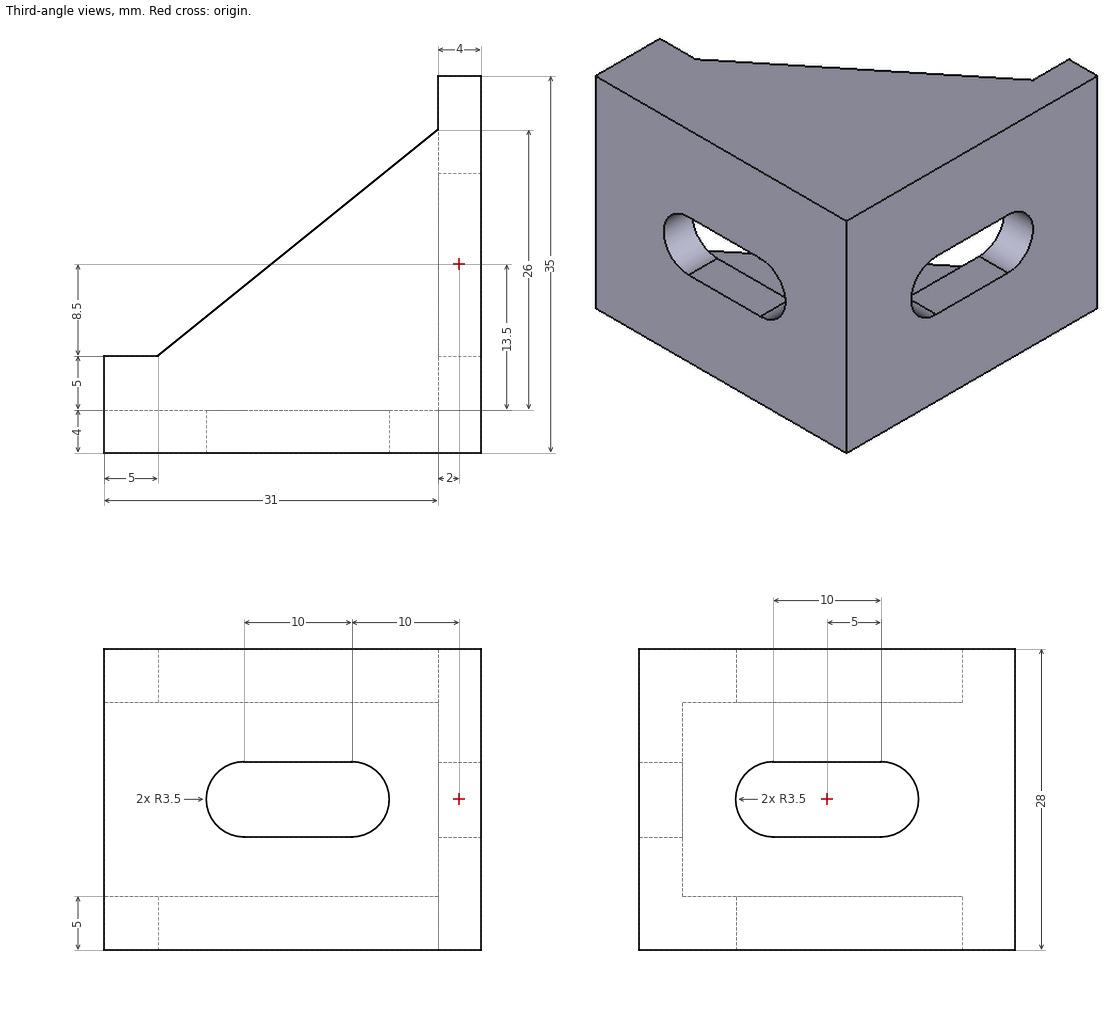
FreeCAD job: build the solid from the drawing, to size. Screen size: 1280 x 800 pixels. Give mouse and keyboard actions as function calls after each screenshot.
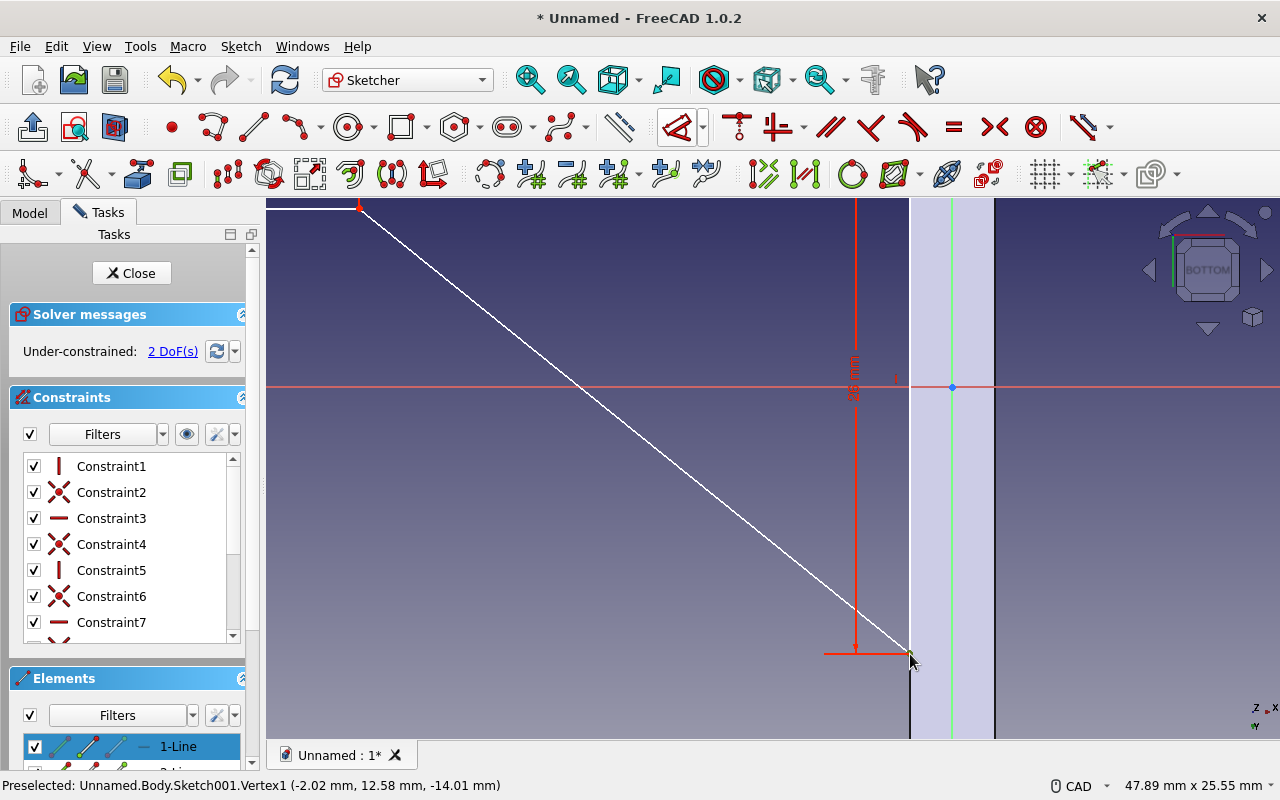
key(l)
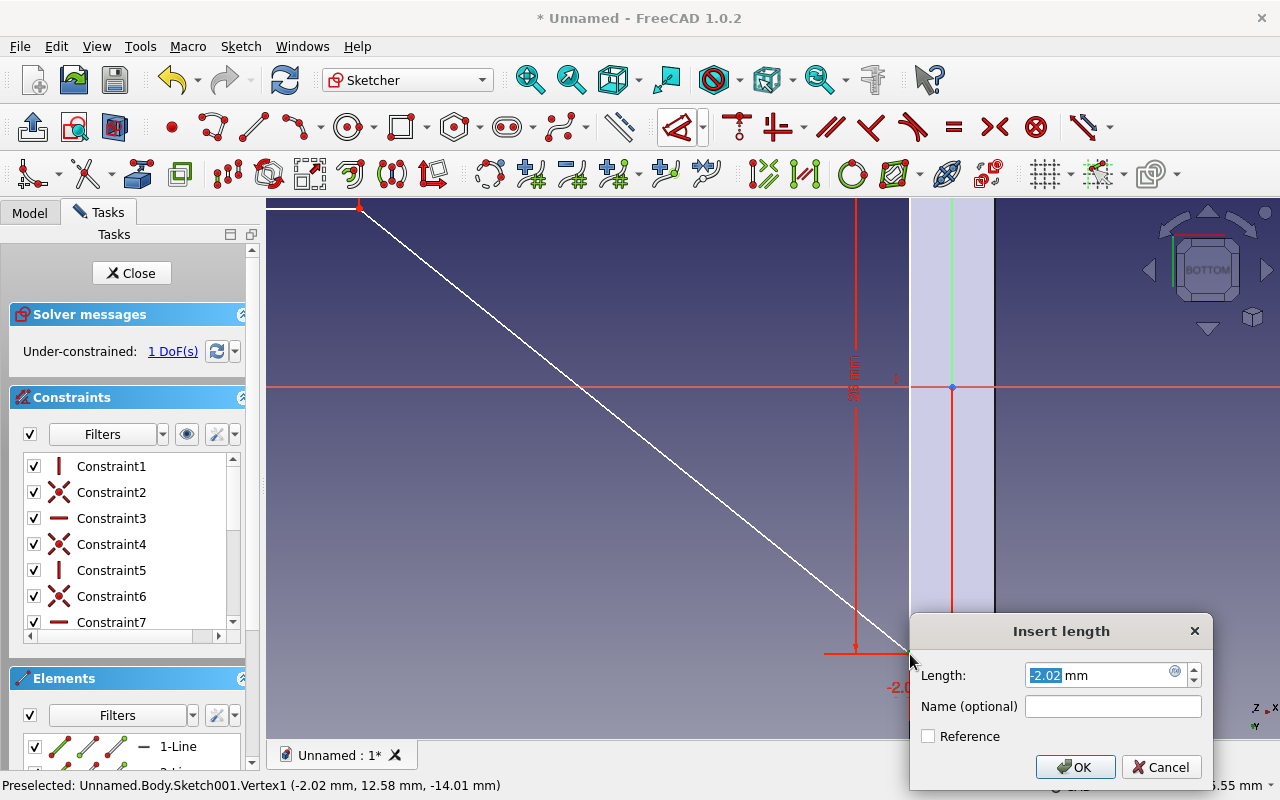
text(-2)
key(Return)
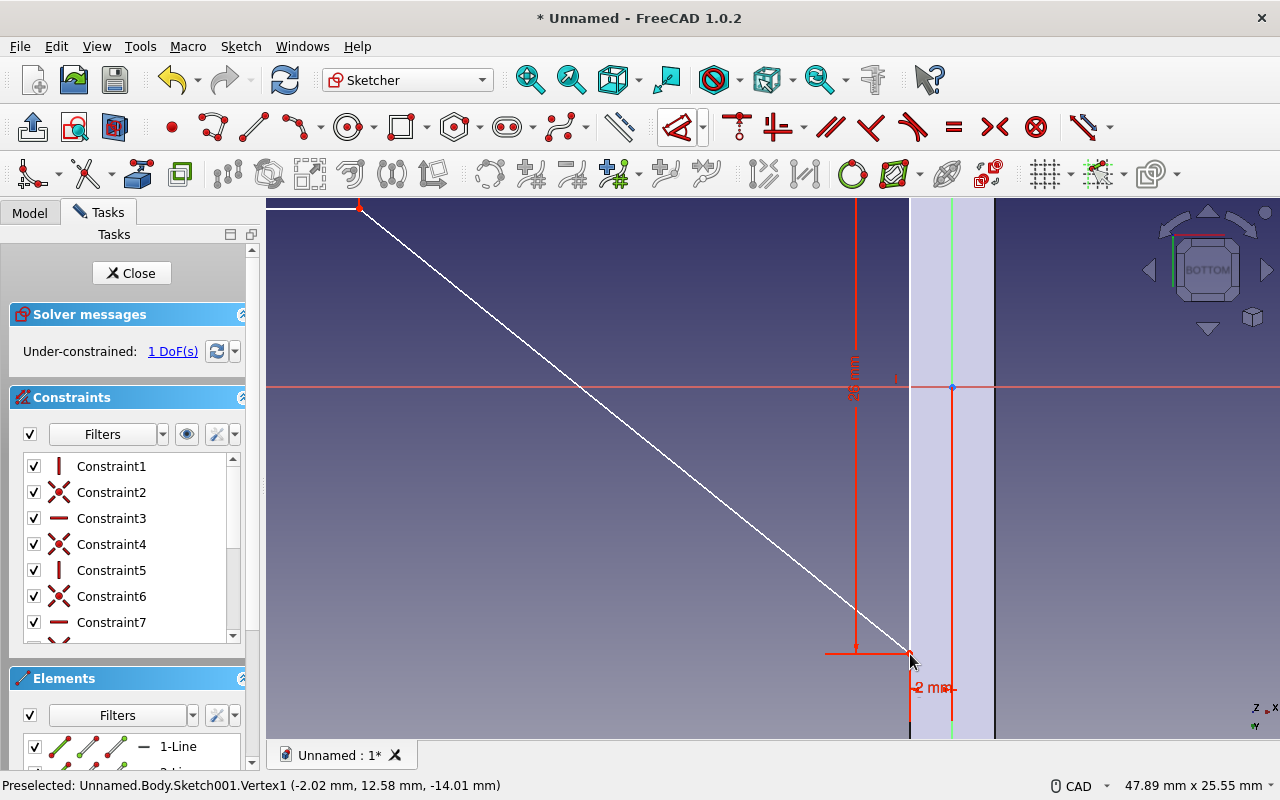
scroll(911, 655, down, 2)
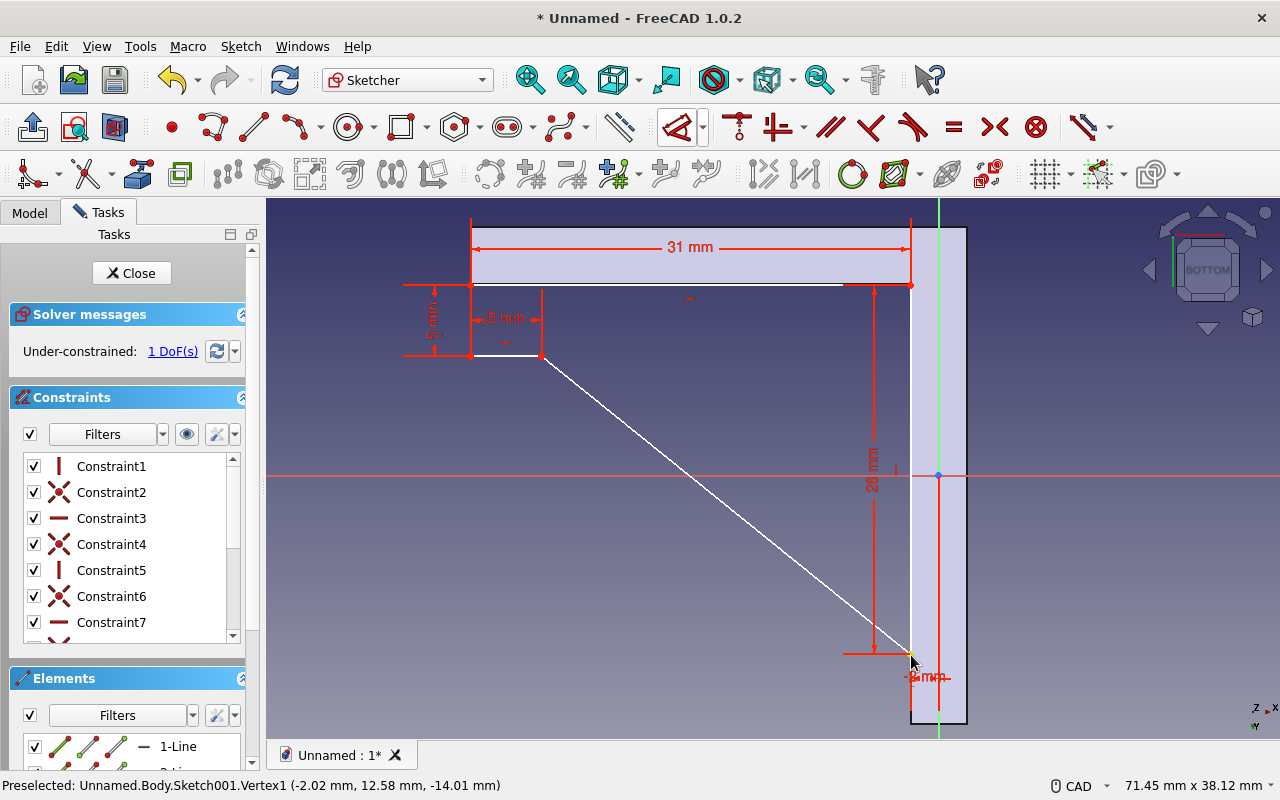
click(471, 356)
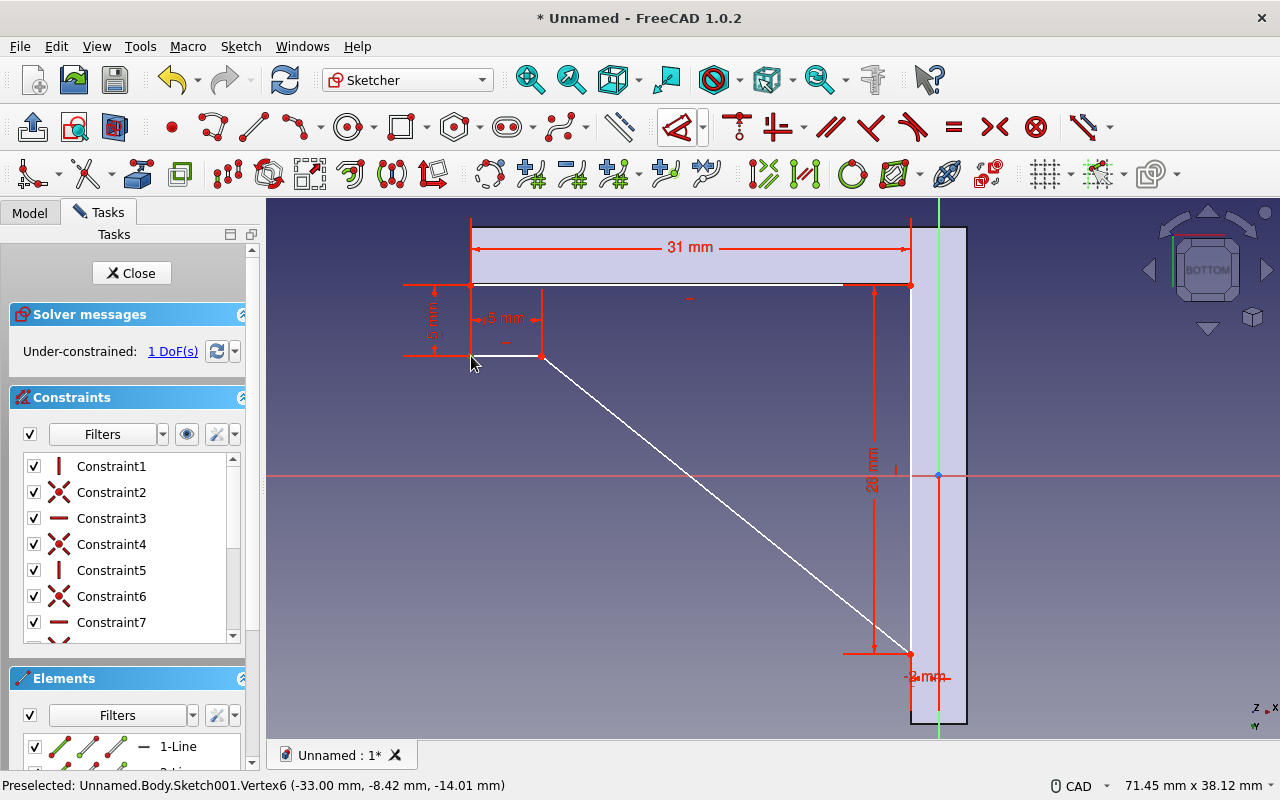
click(702, 128)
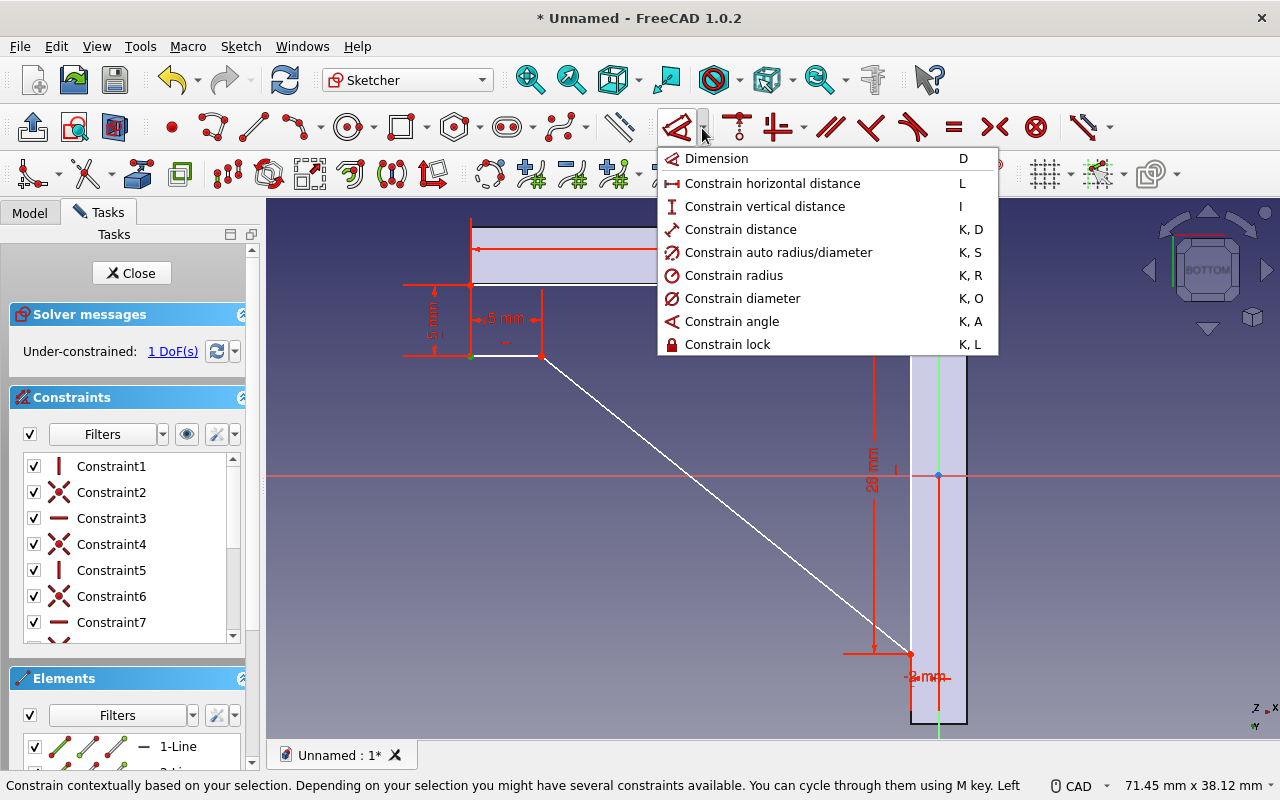
click(828, 206)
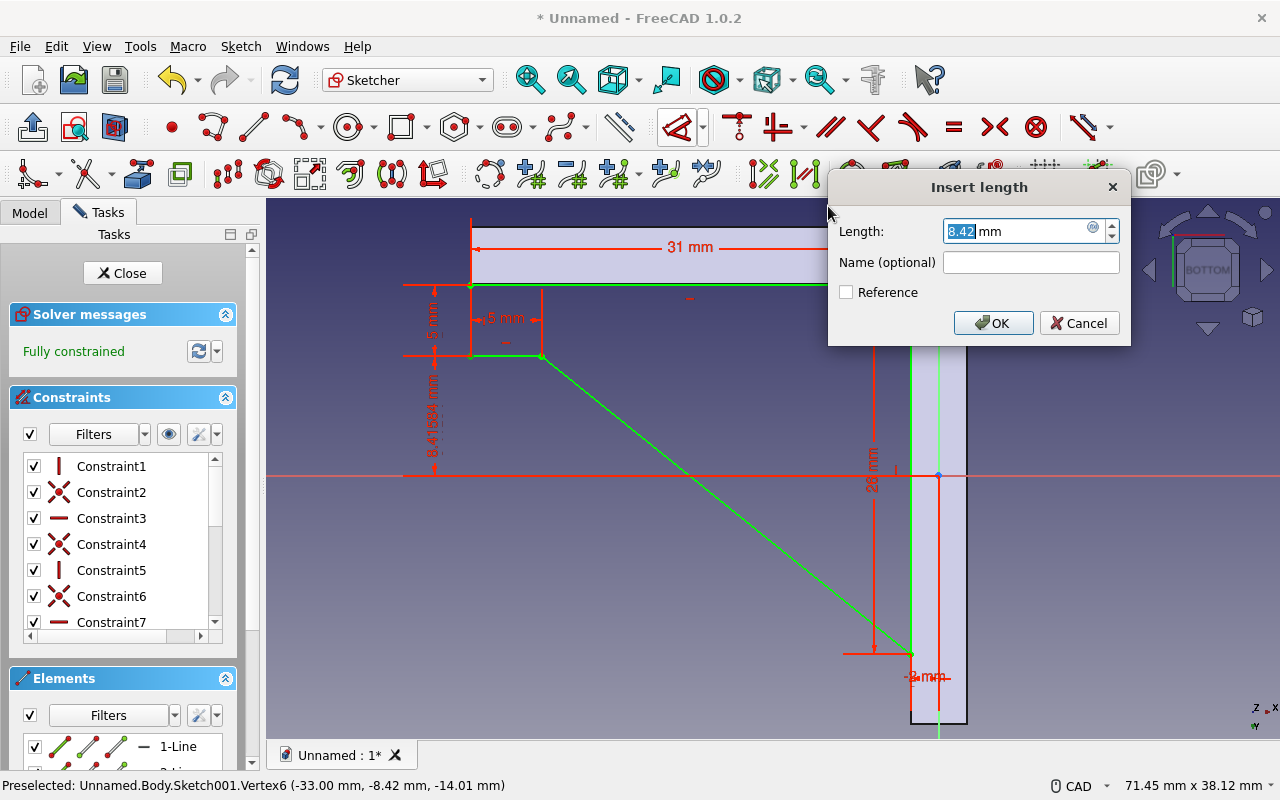
text(8.5)
key(Return)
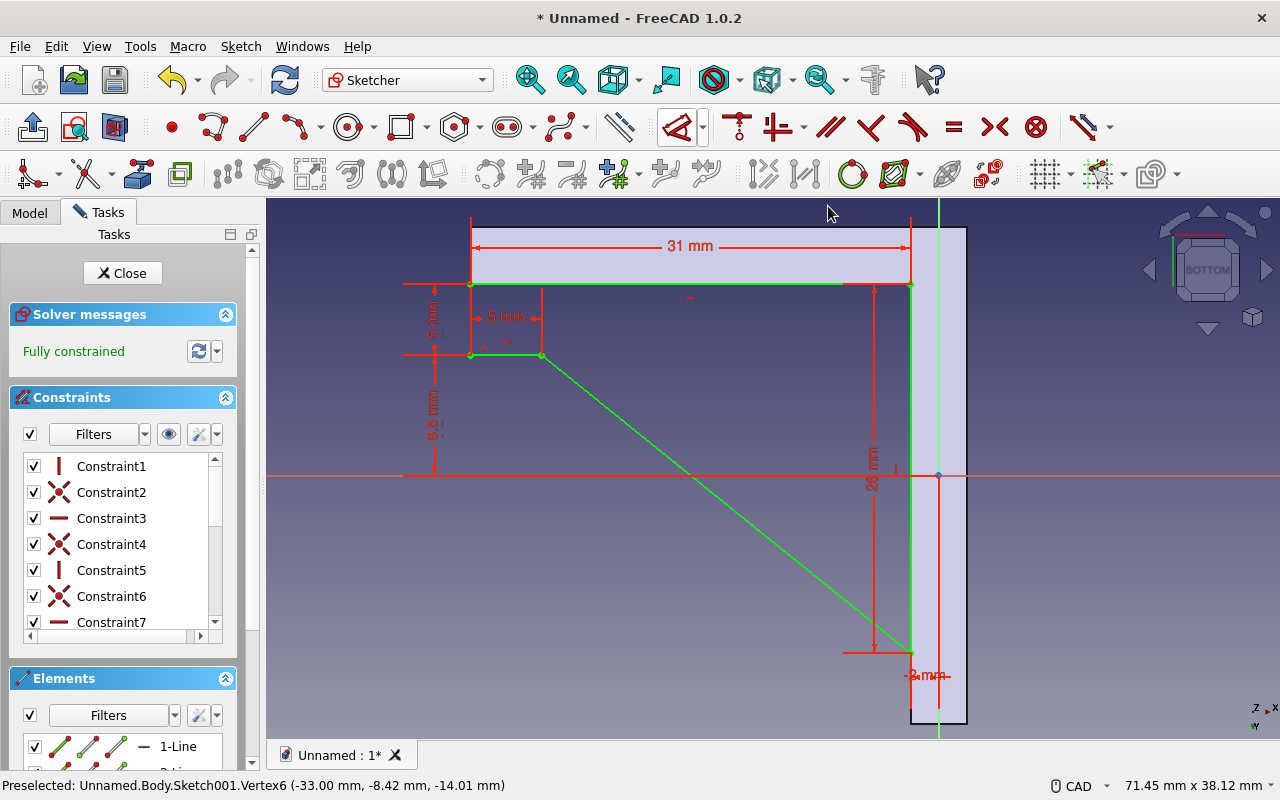
click(123, 273)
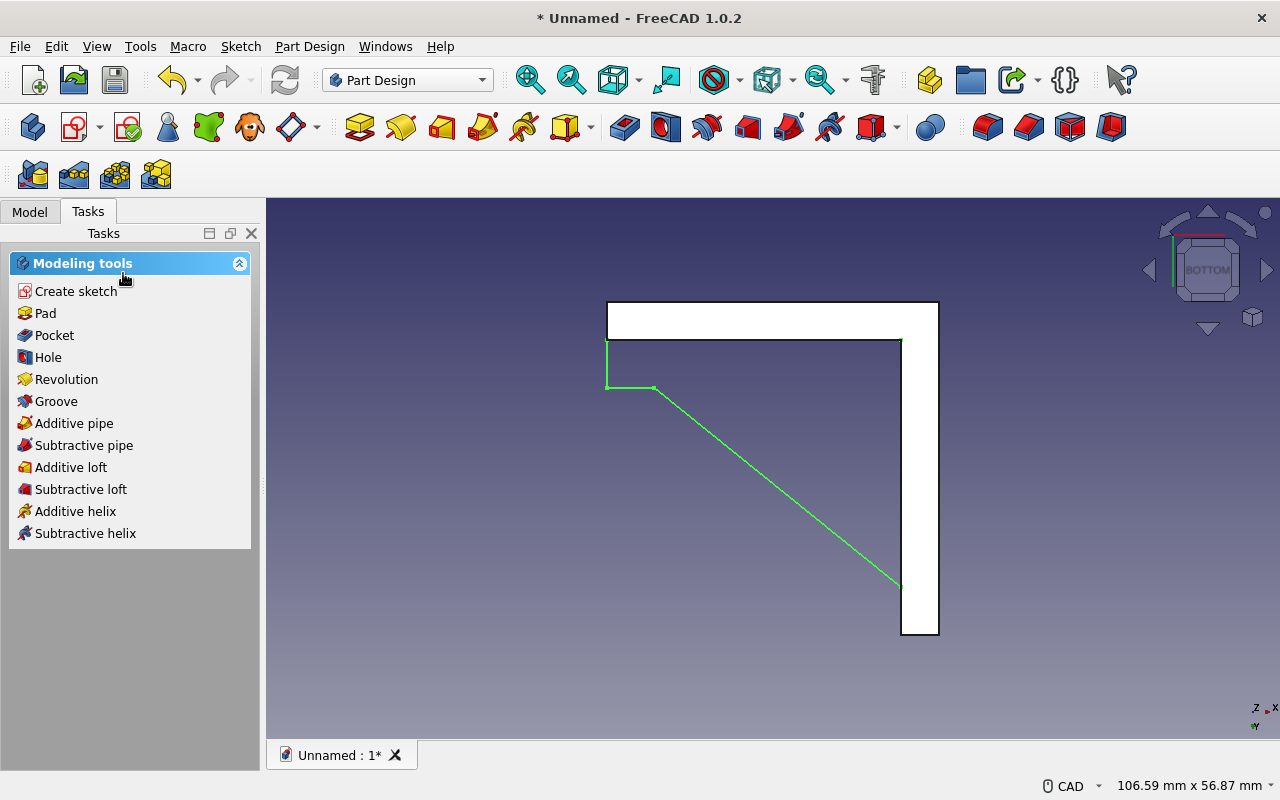
click(360, 128)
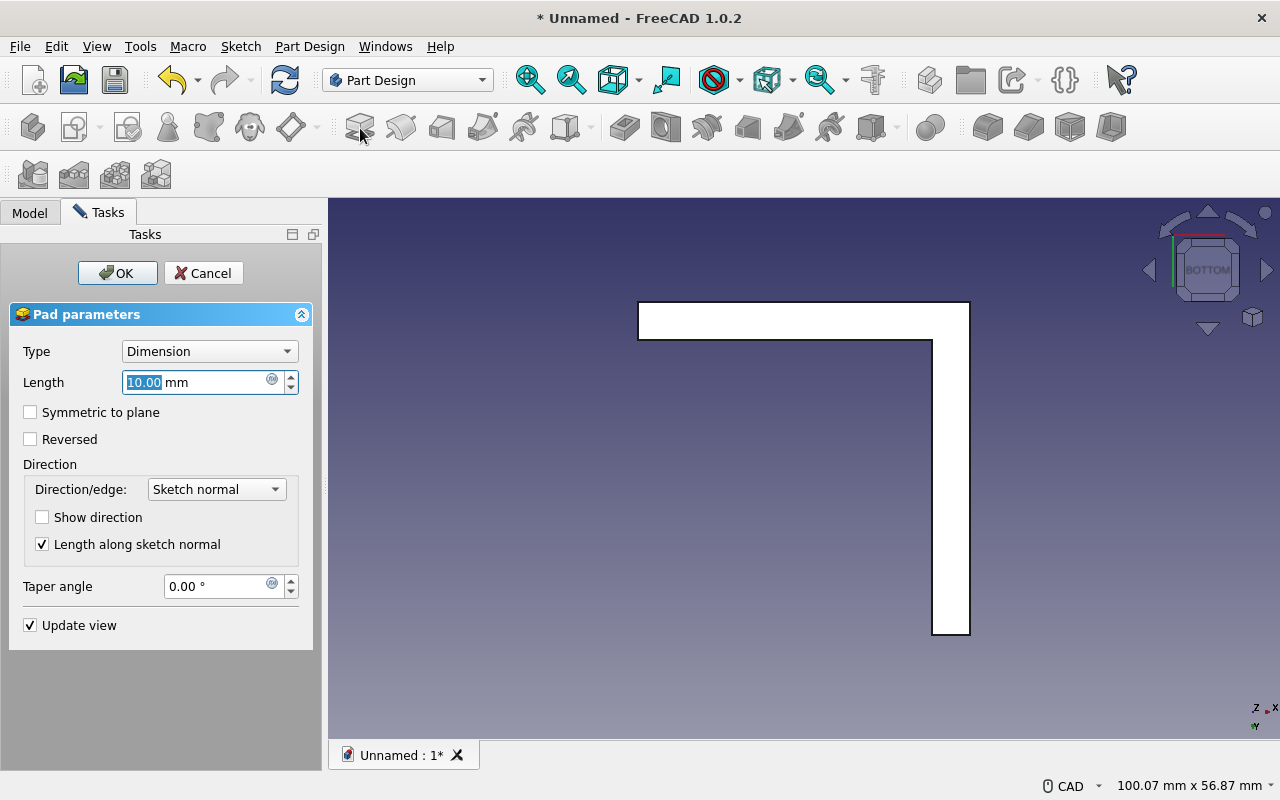
text(5)
key(Tab)